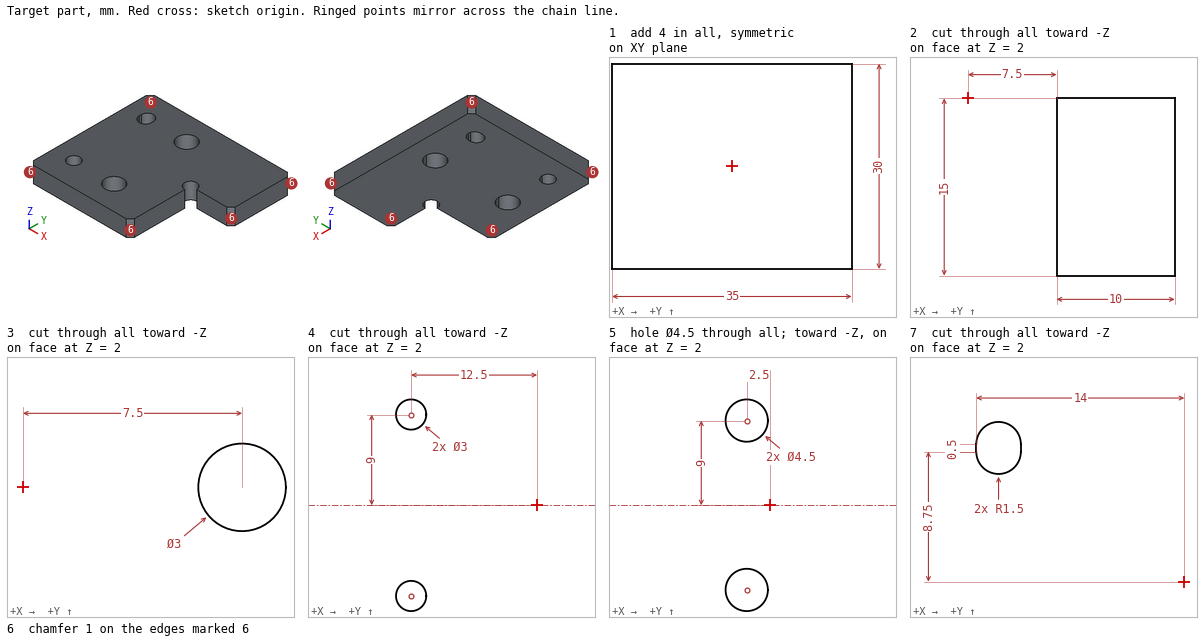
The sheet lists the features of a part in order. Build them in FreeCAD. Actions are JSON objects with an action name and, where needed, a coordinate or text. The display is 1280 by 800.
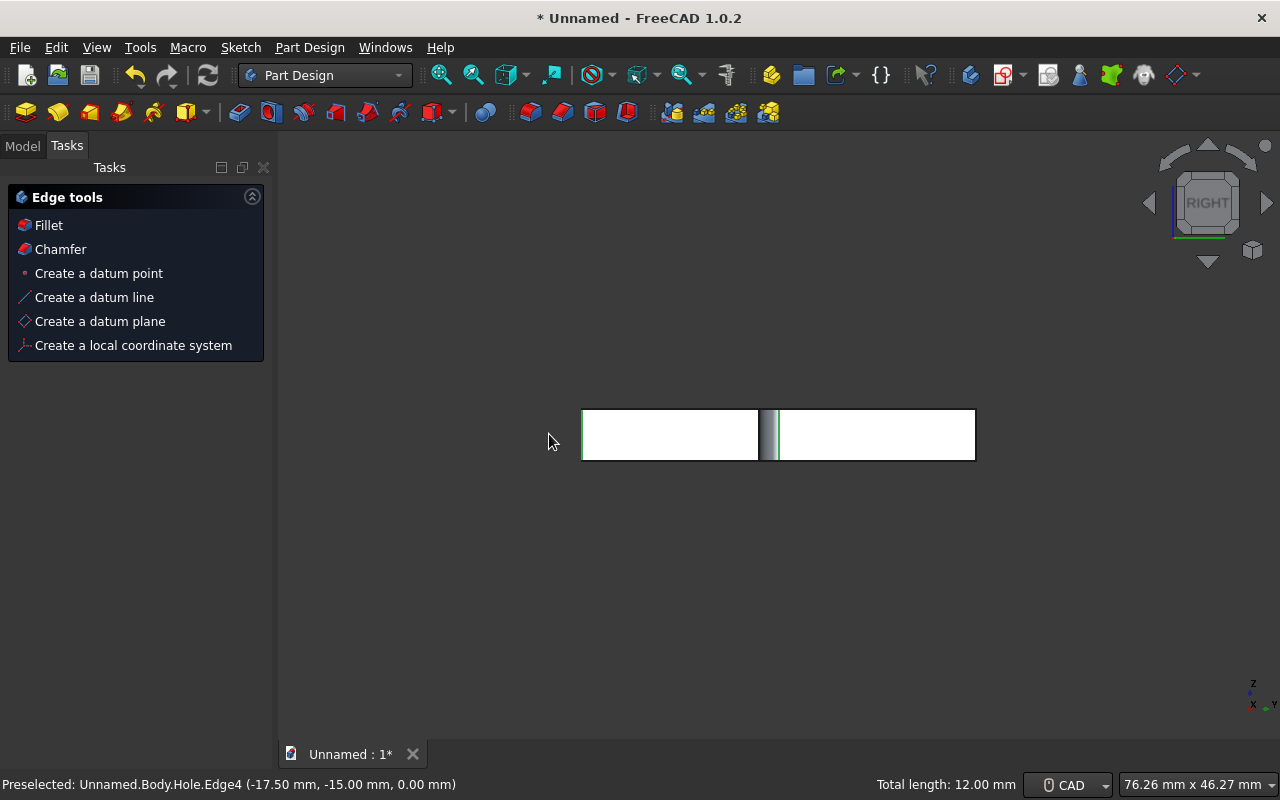
{"action": "left_click", "coordinate": [976, 434], "text": "ctrl"}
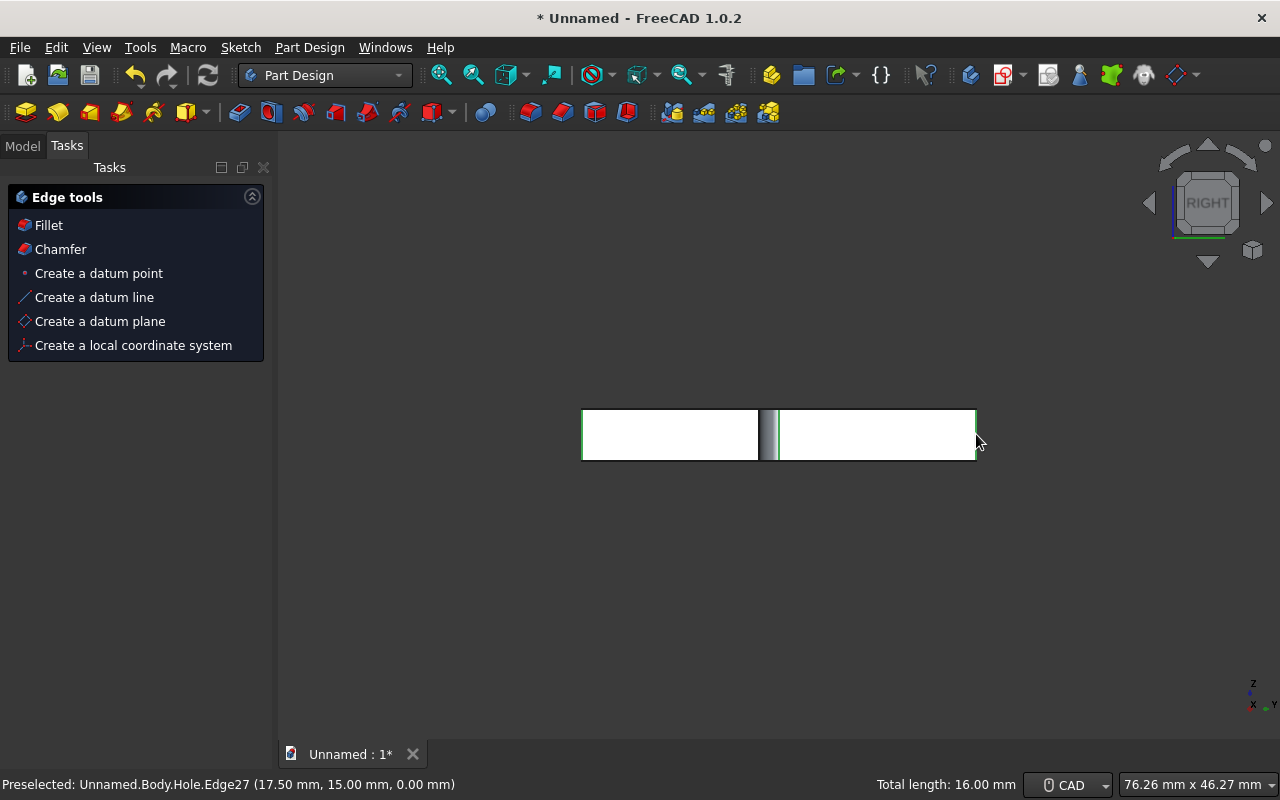
{"action": "key", "text": "5"}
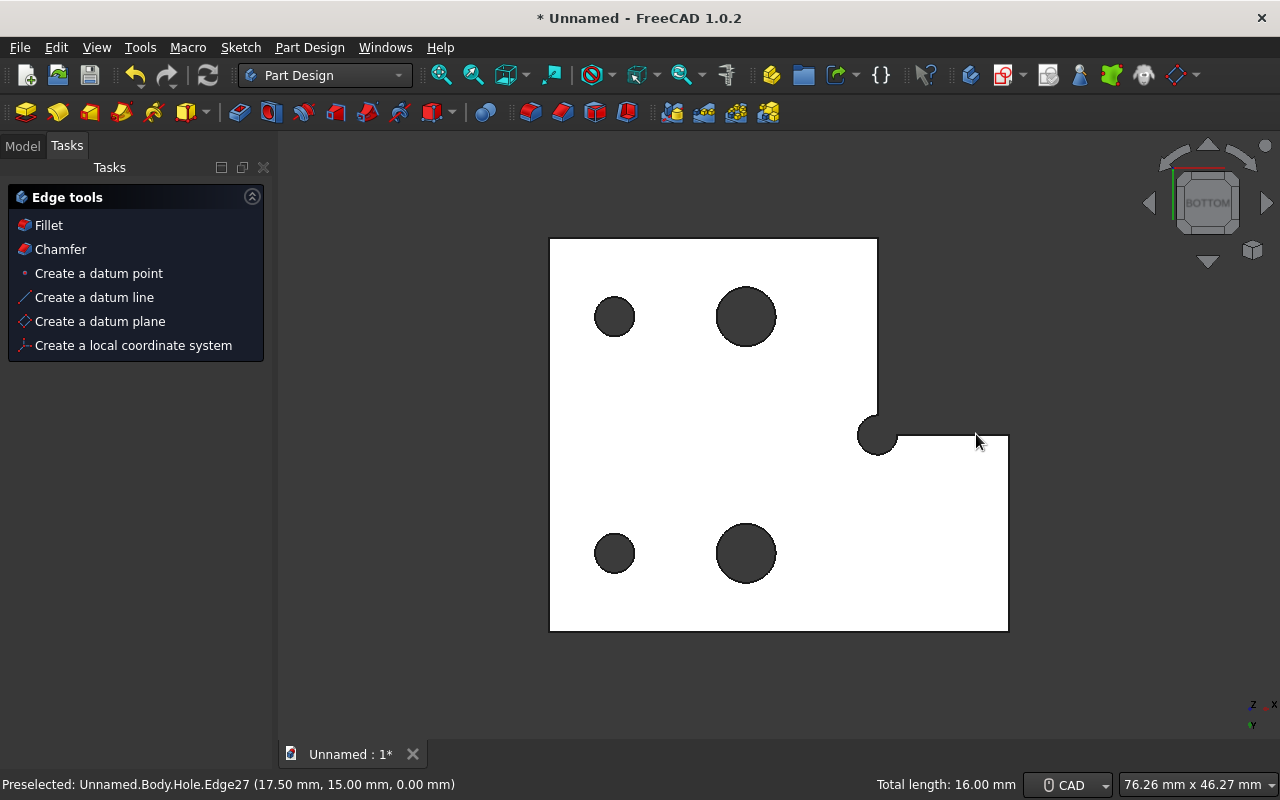
{"action": "key", "text": "4"}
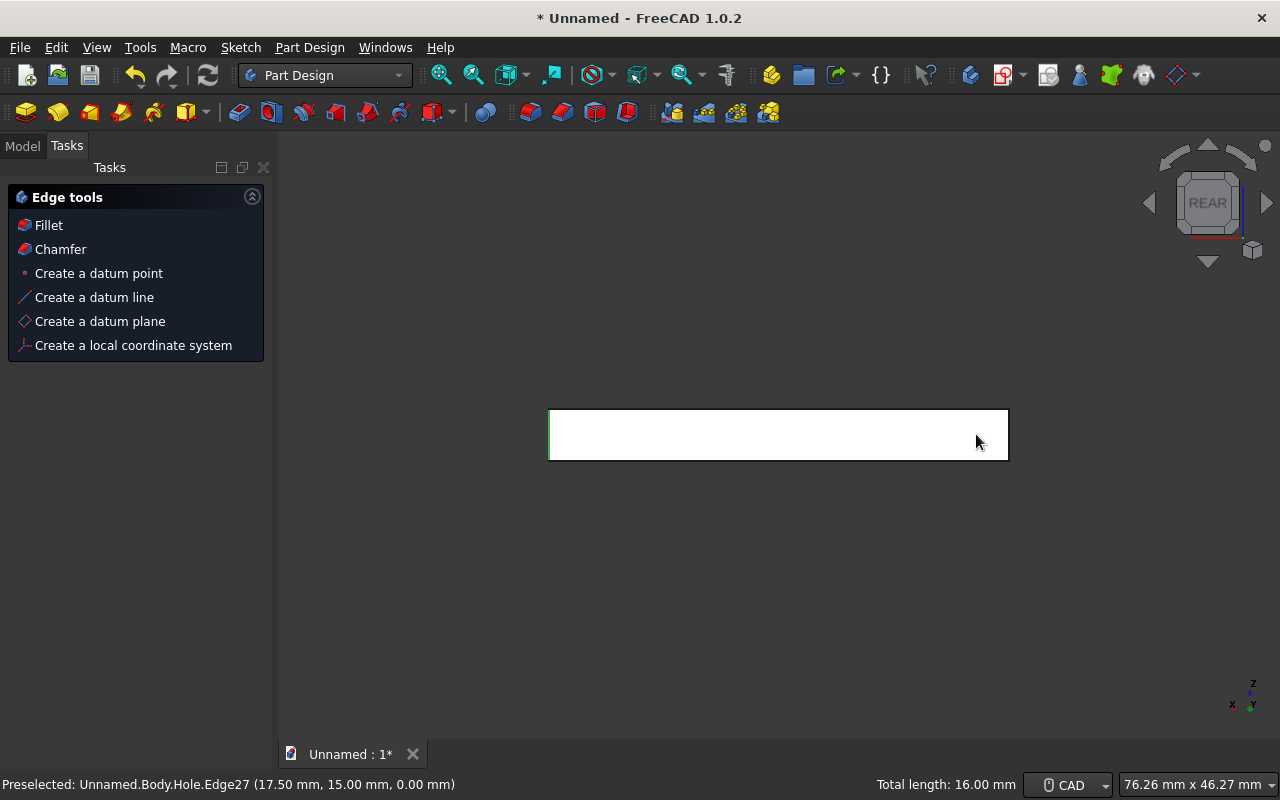
{"action": "left_click", "coordinate": [1009, 434], "text": "ctrl"}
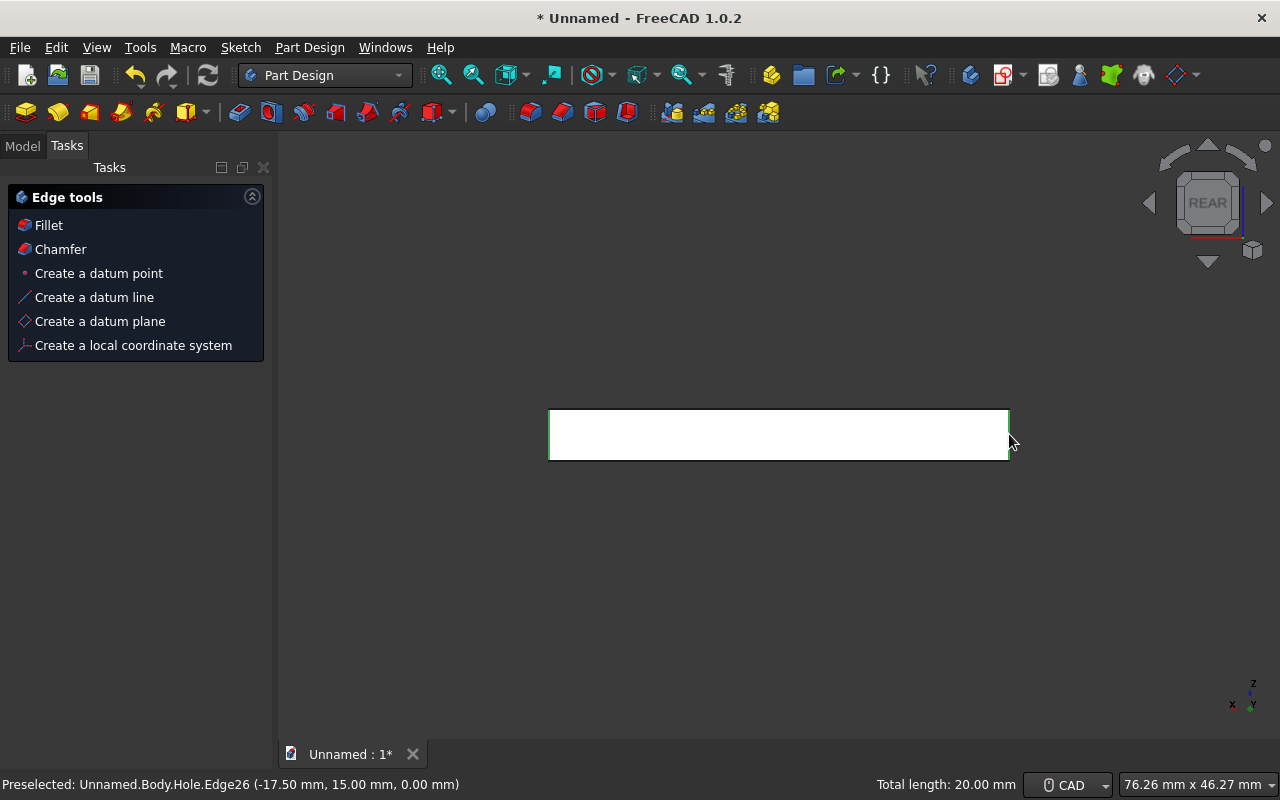
{"action": "left_click", "coordinate": [564, 112]}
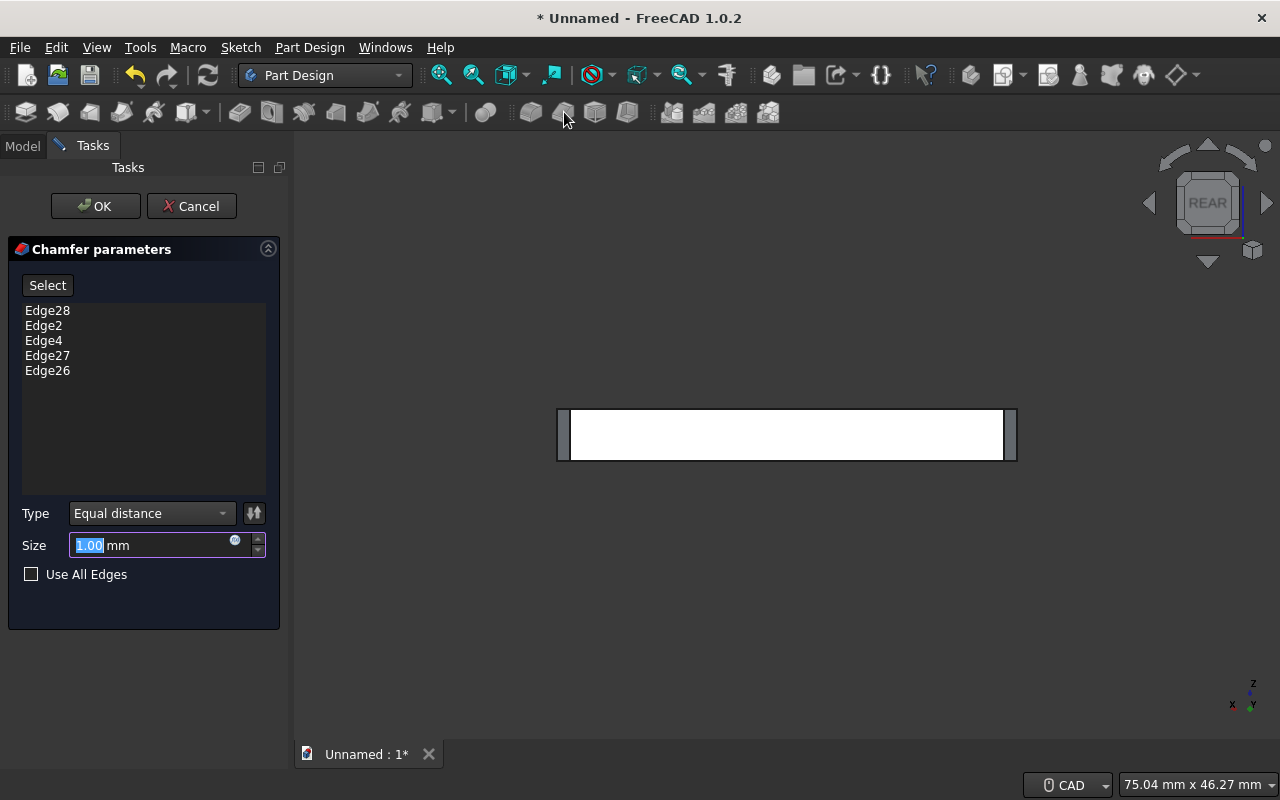
{"action": "type", "text": "1"}
{"action": "key", "text": "Tab"}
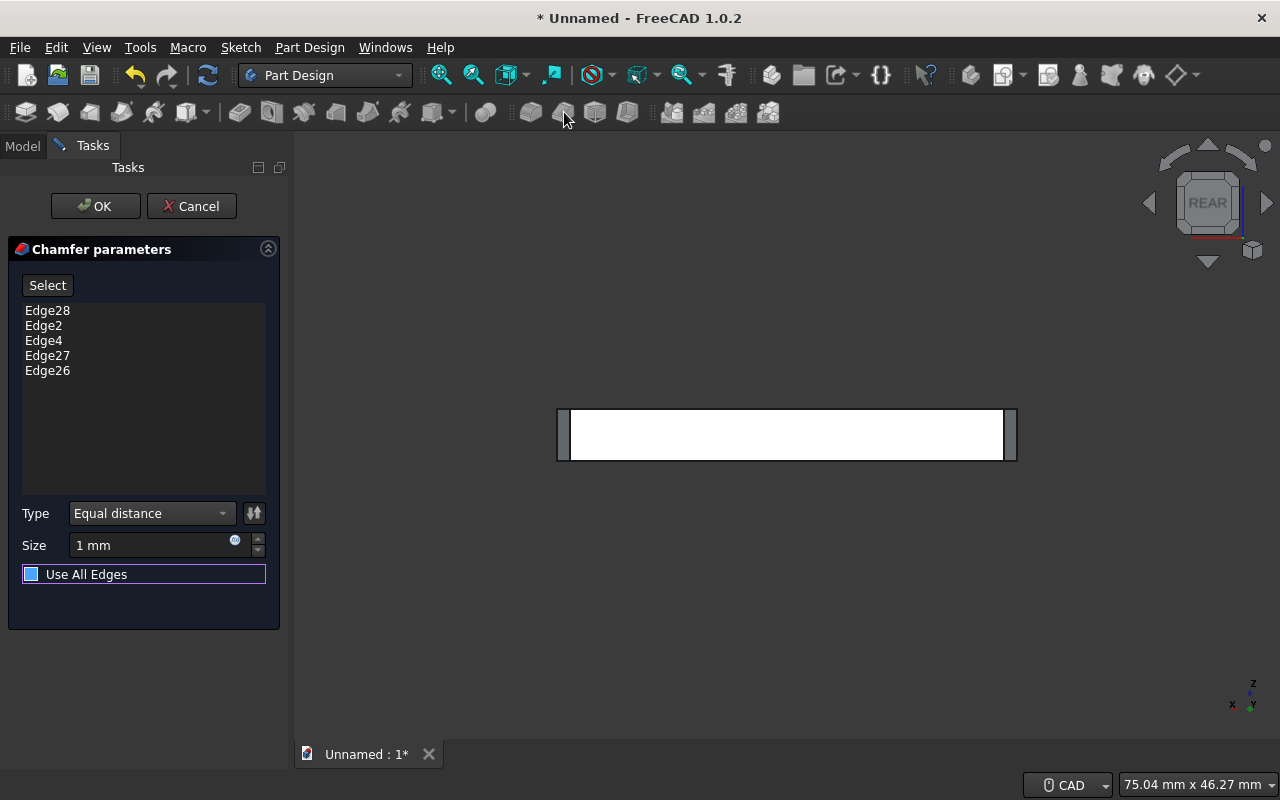
{"action": "left_click", "coordinate": [96, 206]}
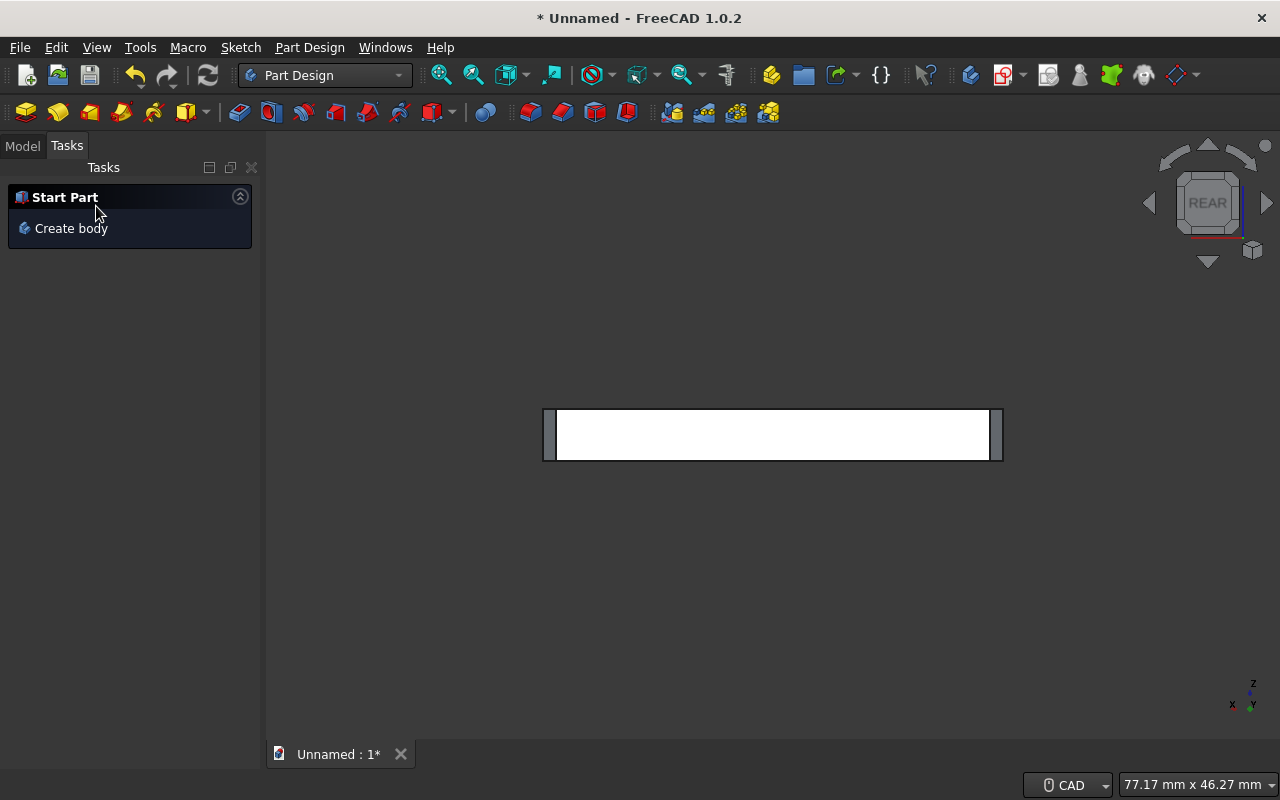
{"action": "key", "text": "0"}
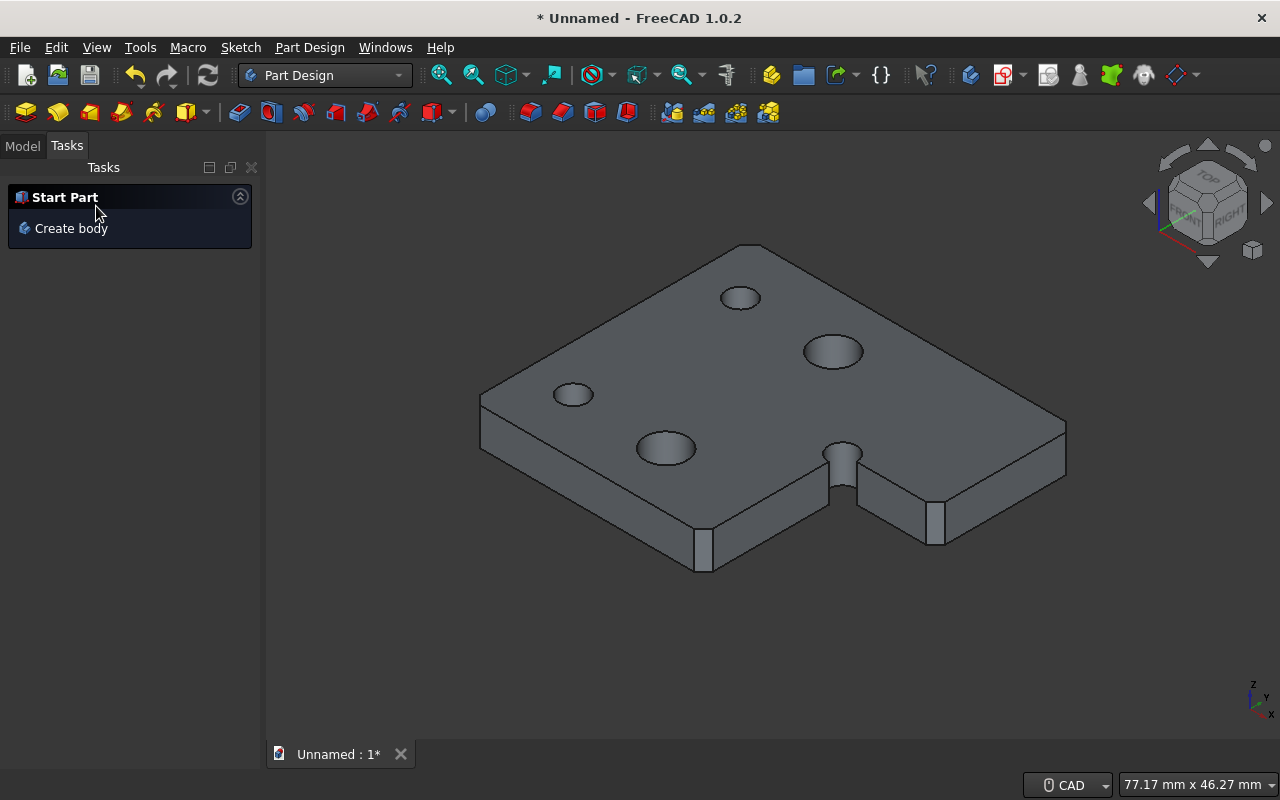
{"action": "left_click", "coordinate": [680, 359]}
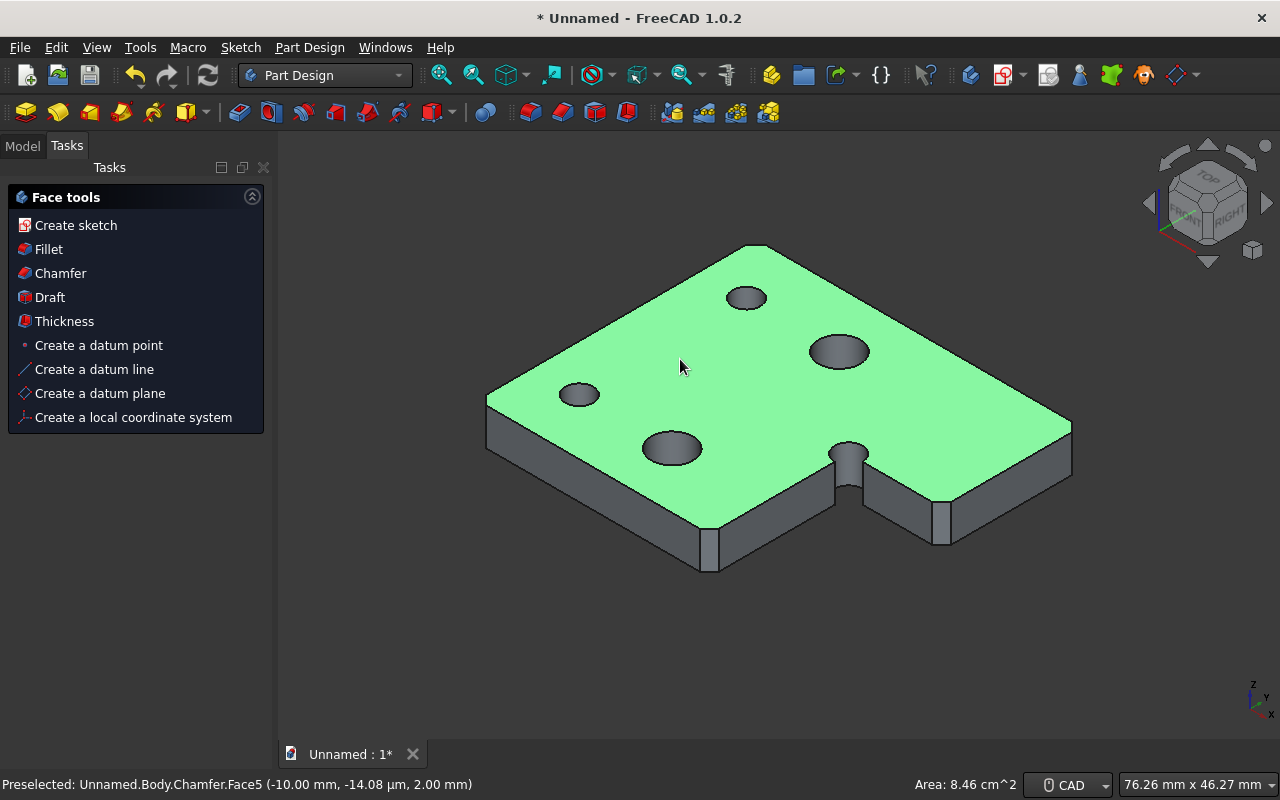
{"action": "left_click", "coordinate": [1004, 76]}